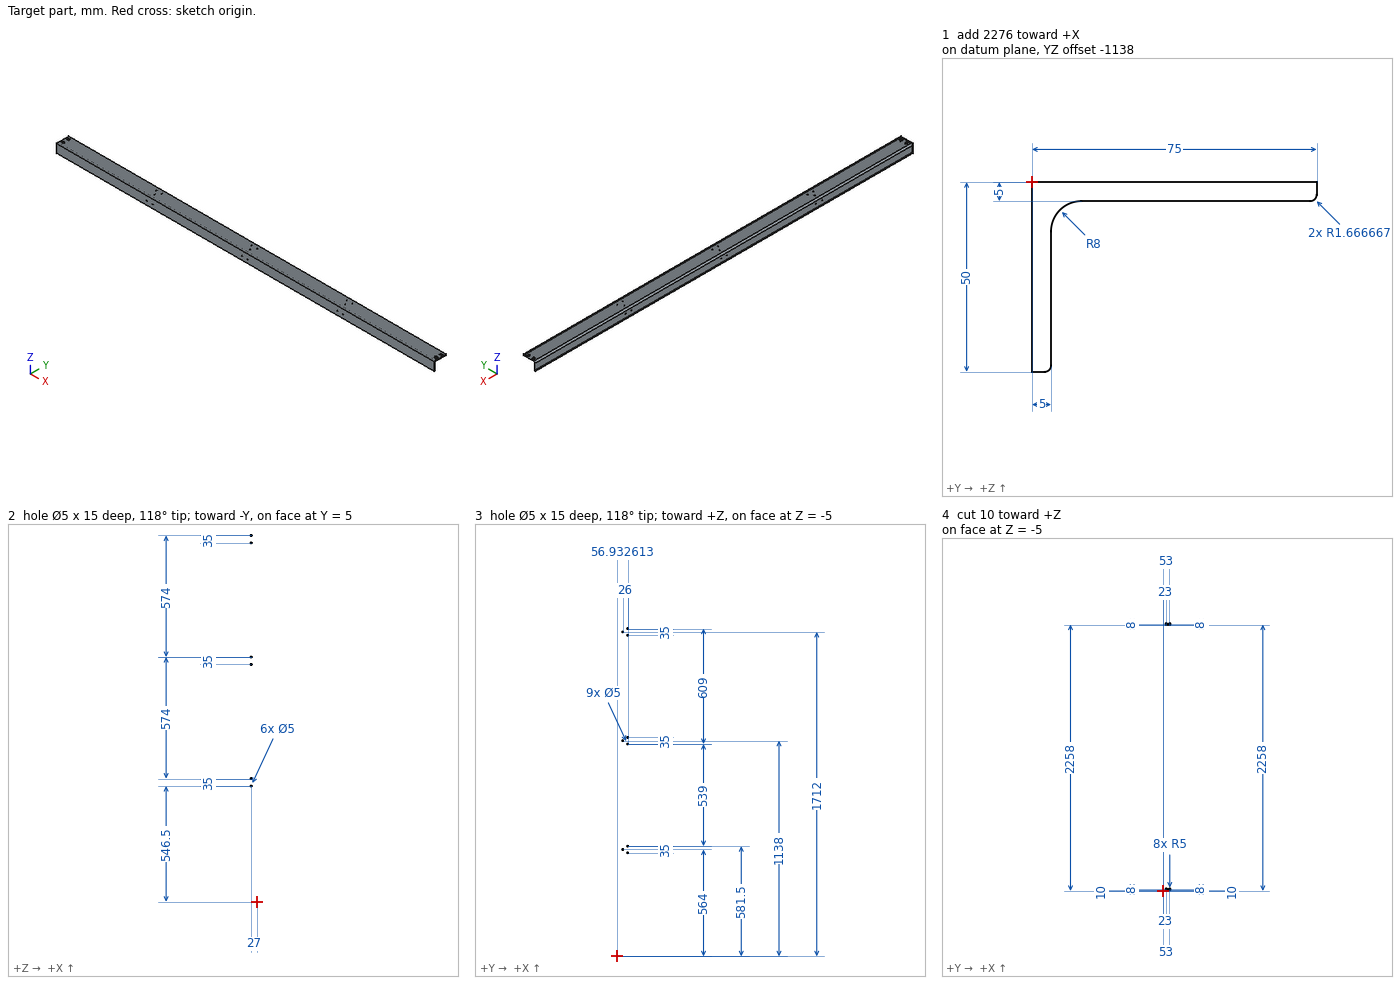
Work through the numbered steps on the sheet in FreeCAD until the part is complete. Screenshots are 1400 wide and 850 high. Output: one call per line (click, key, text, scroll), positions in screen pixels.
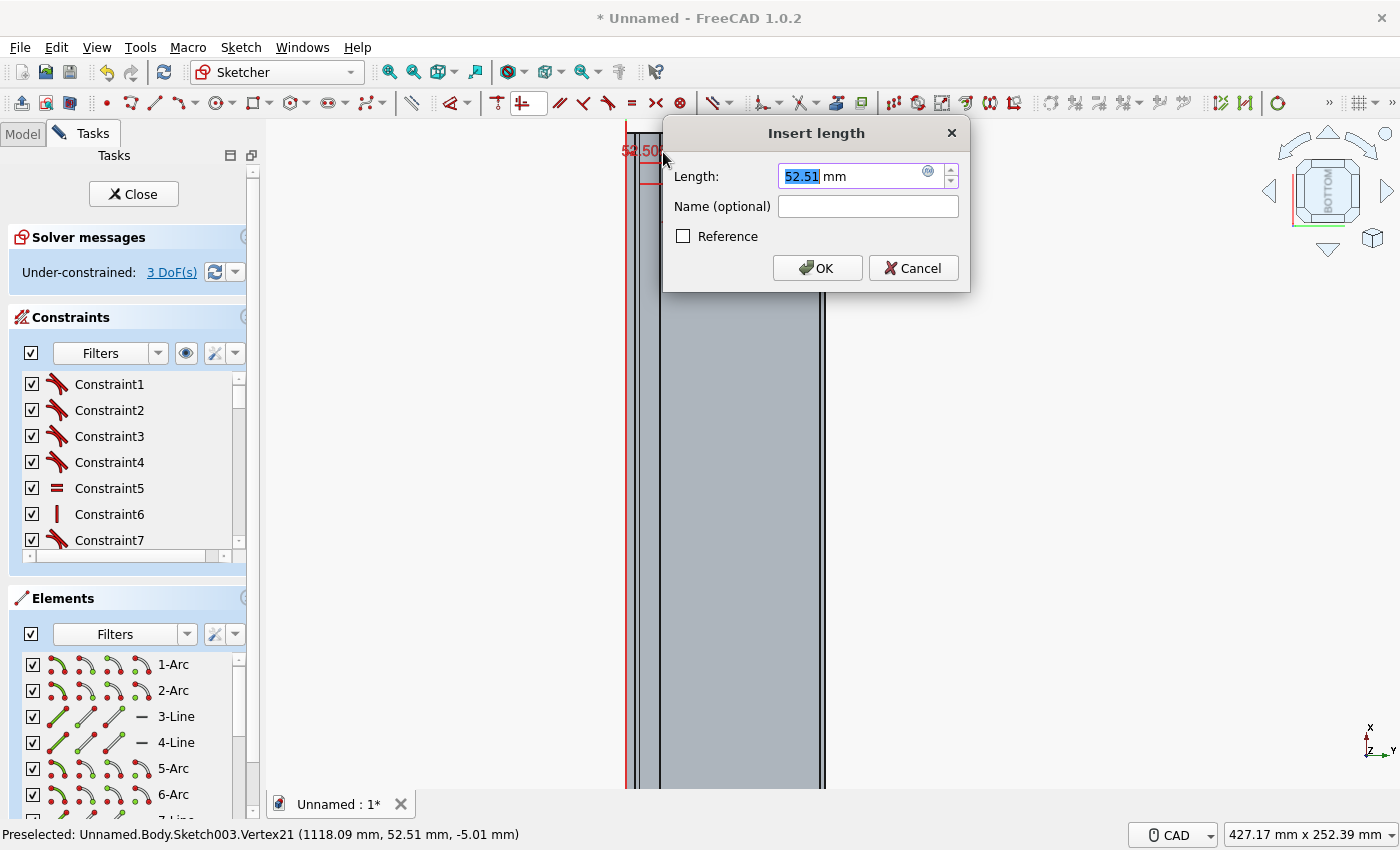
text(53)
key(Return)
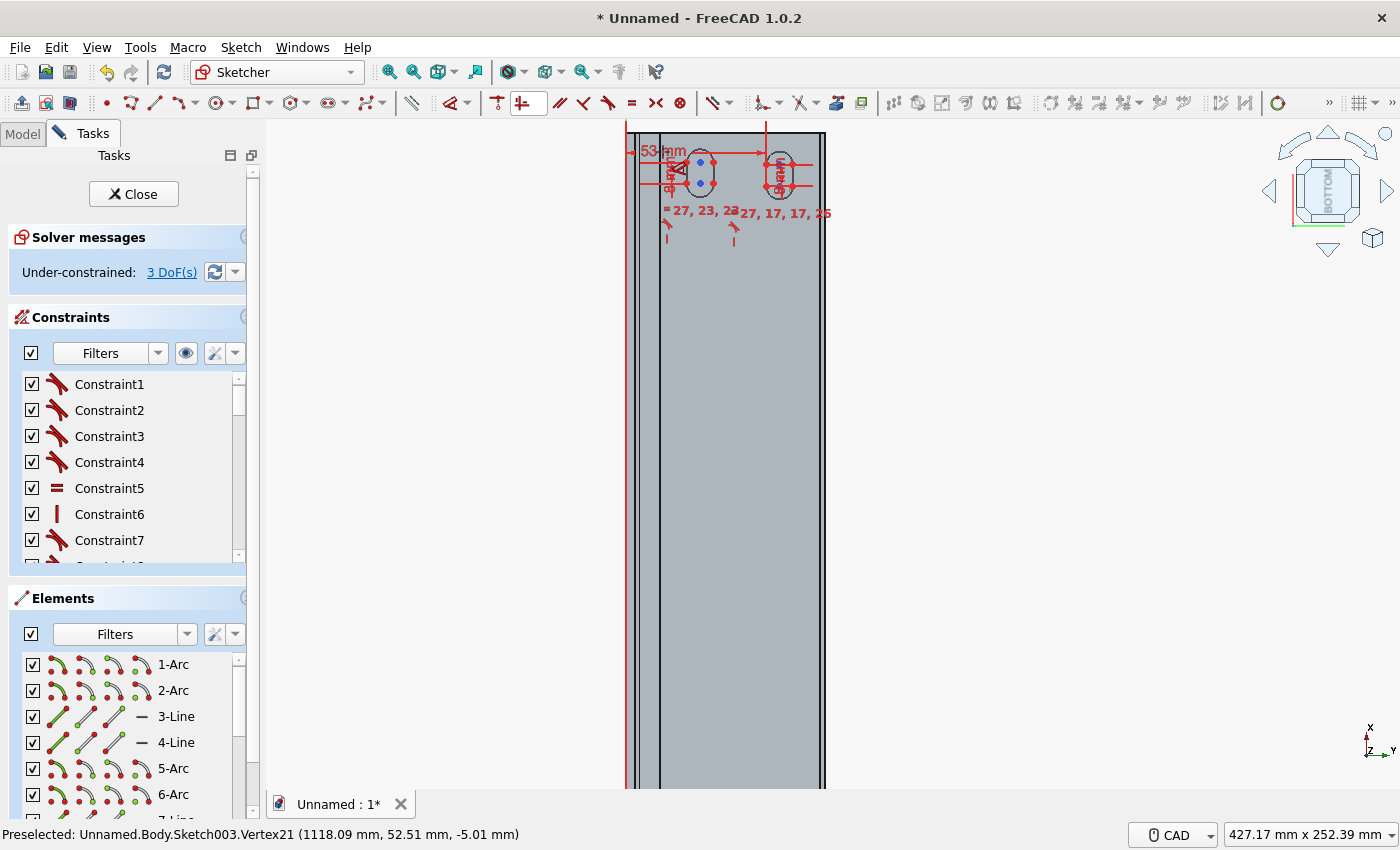
click(687, 184)
click(656, 150)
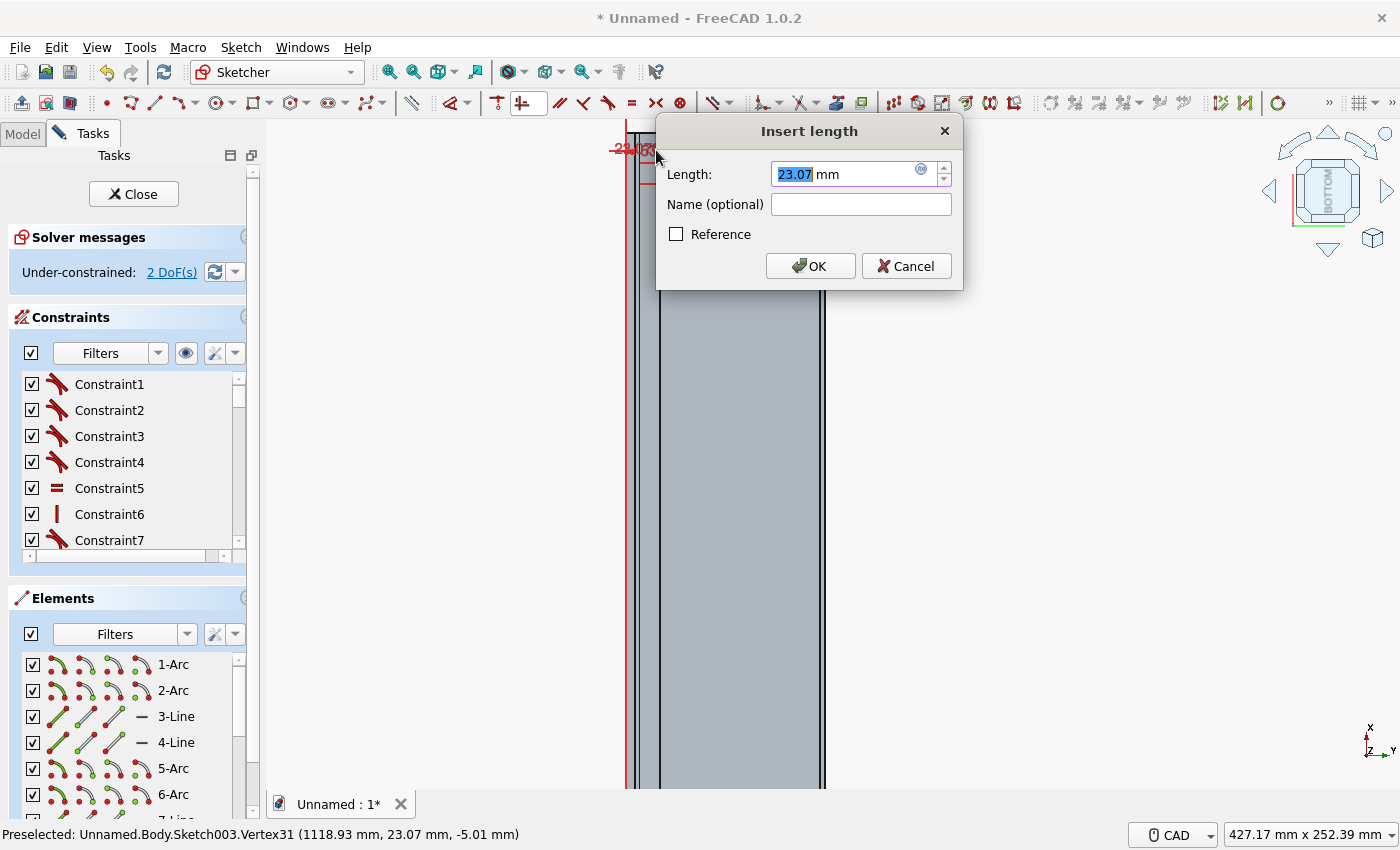
text(23)
key(Return)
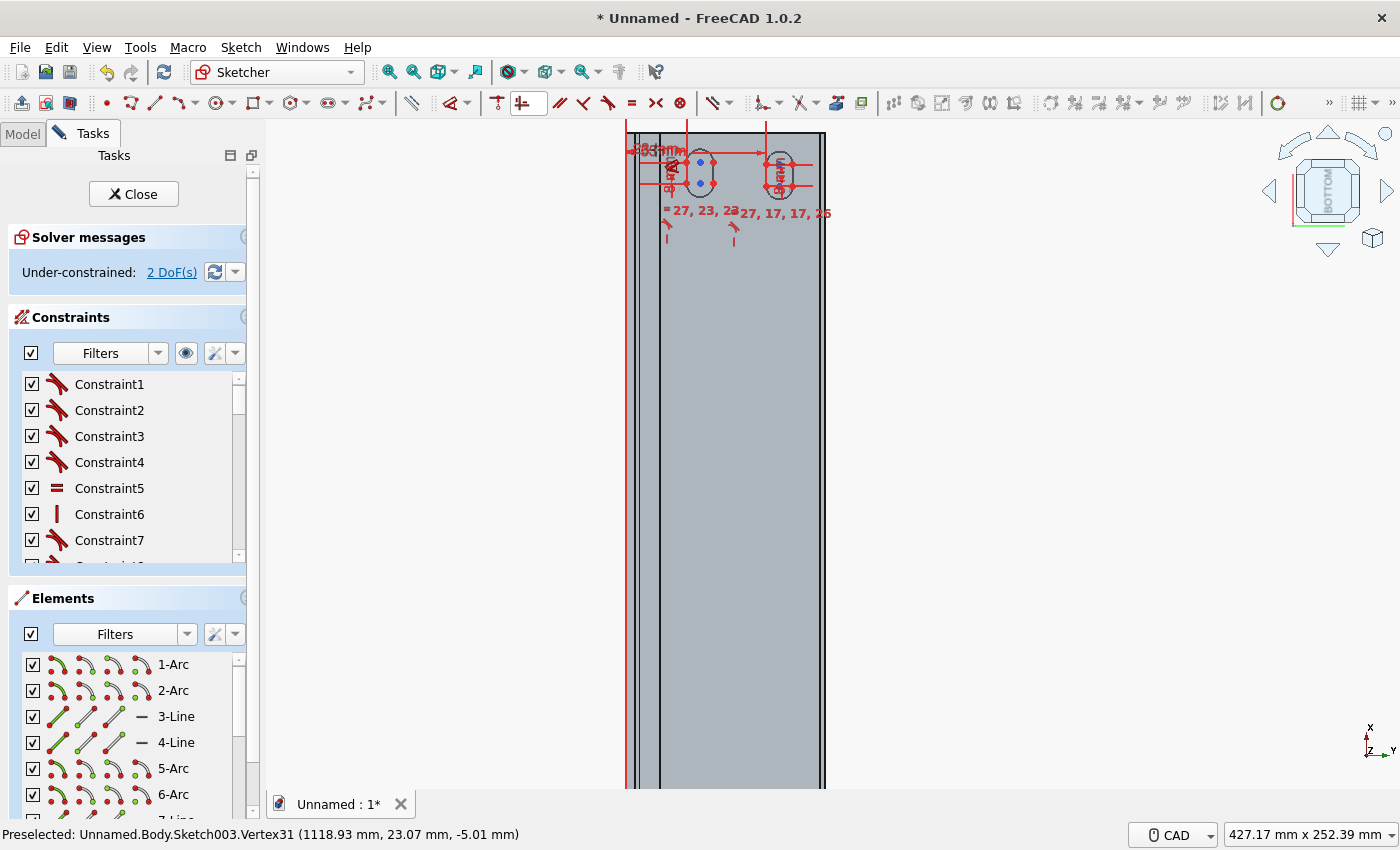
click(766, 186)
click(592, 474)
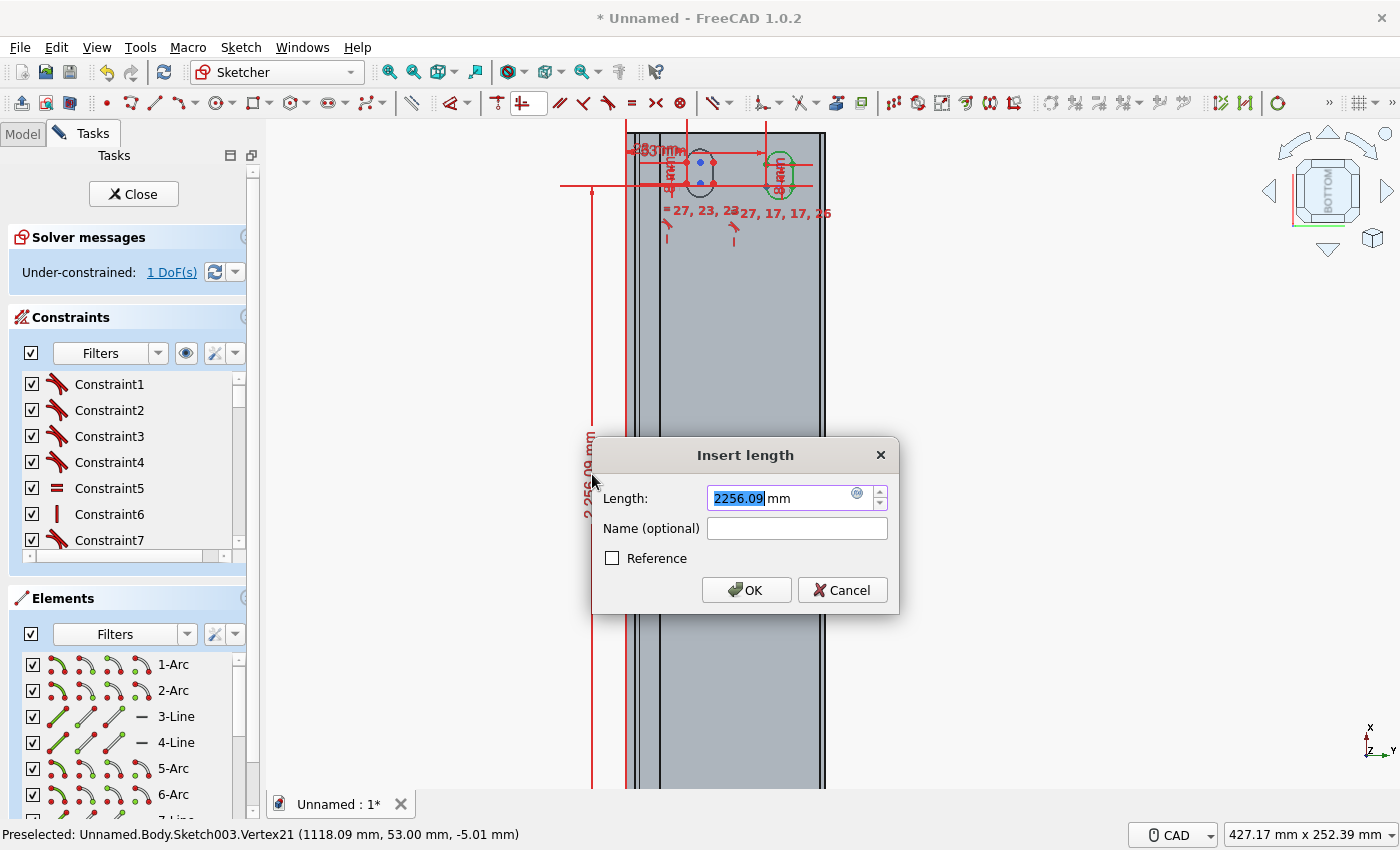
text(2258)
key(Return)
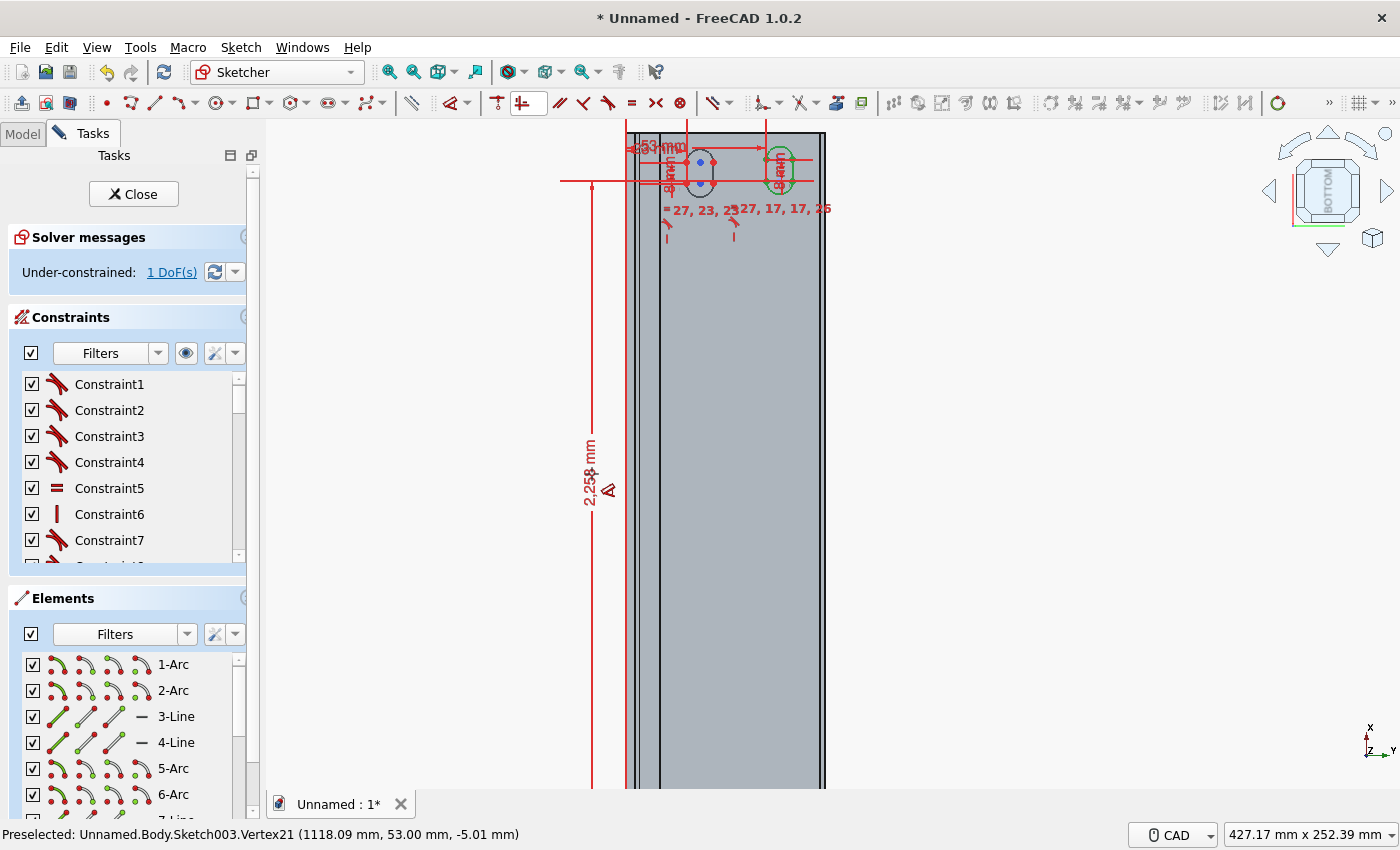
click(687, 184)
click(592, 340)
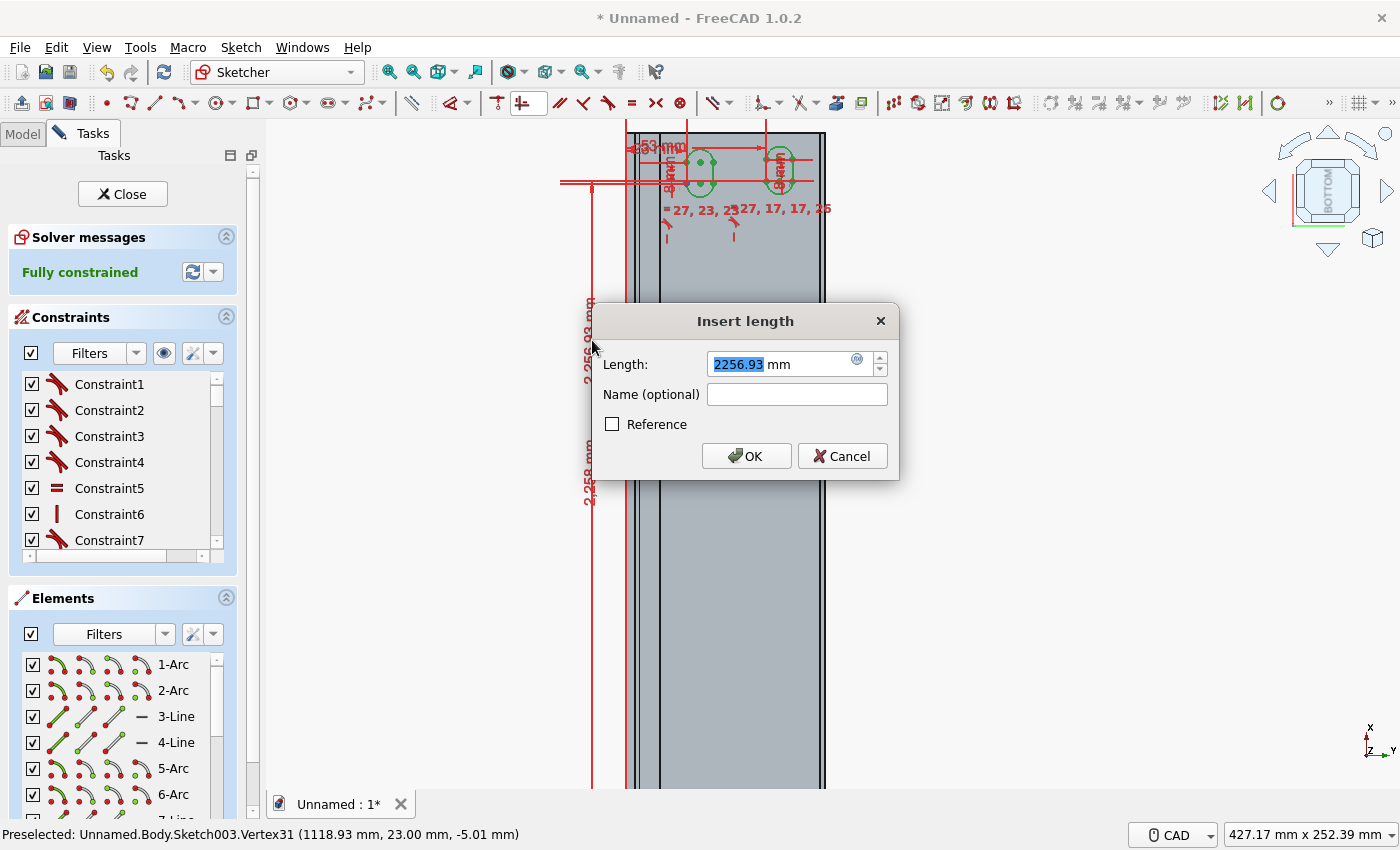
text(2258)
key(Return)
key(Escape)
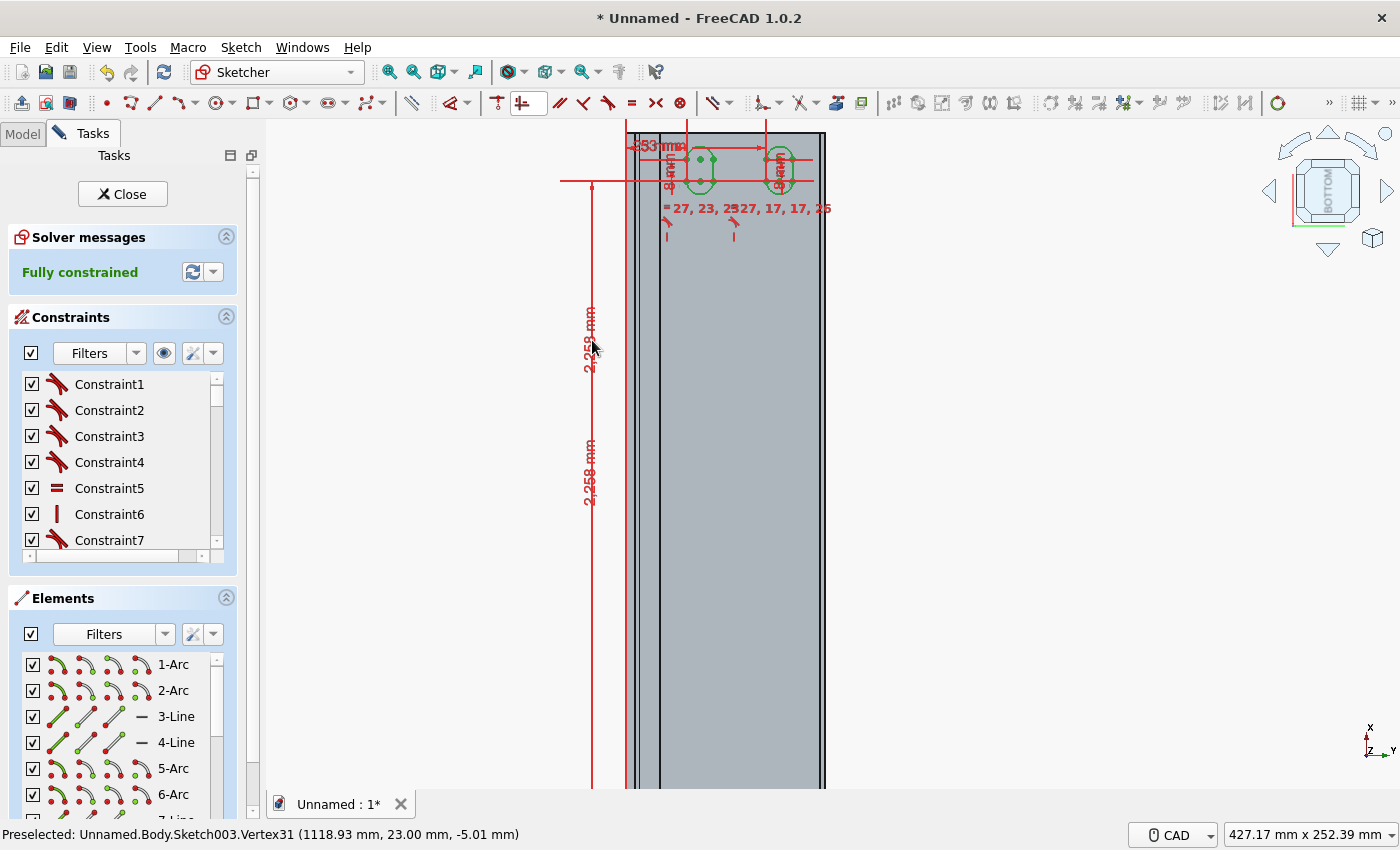
click(123, 194)